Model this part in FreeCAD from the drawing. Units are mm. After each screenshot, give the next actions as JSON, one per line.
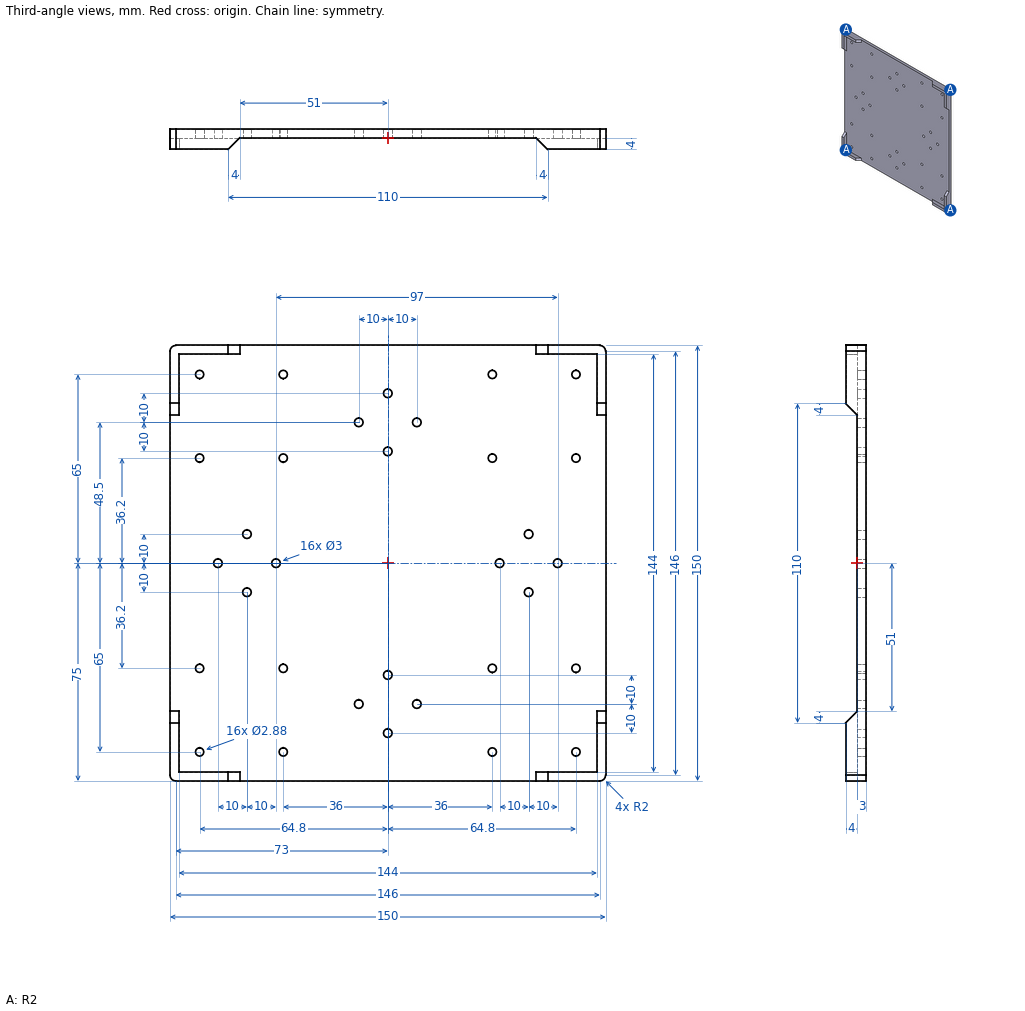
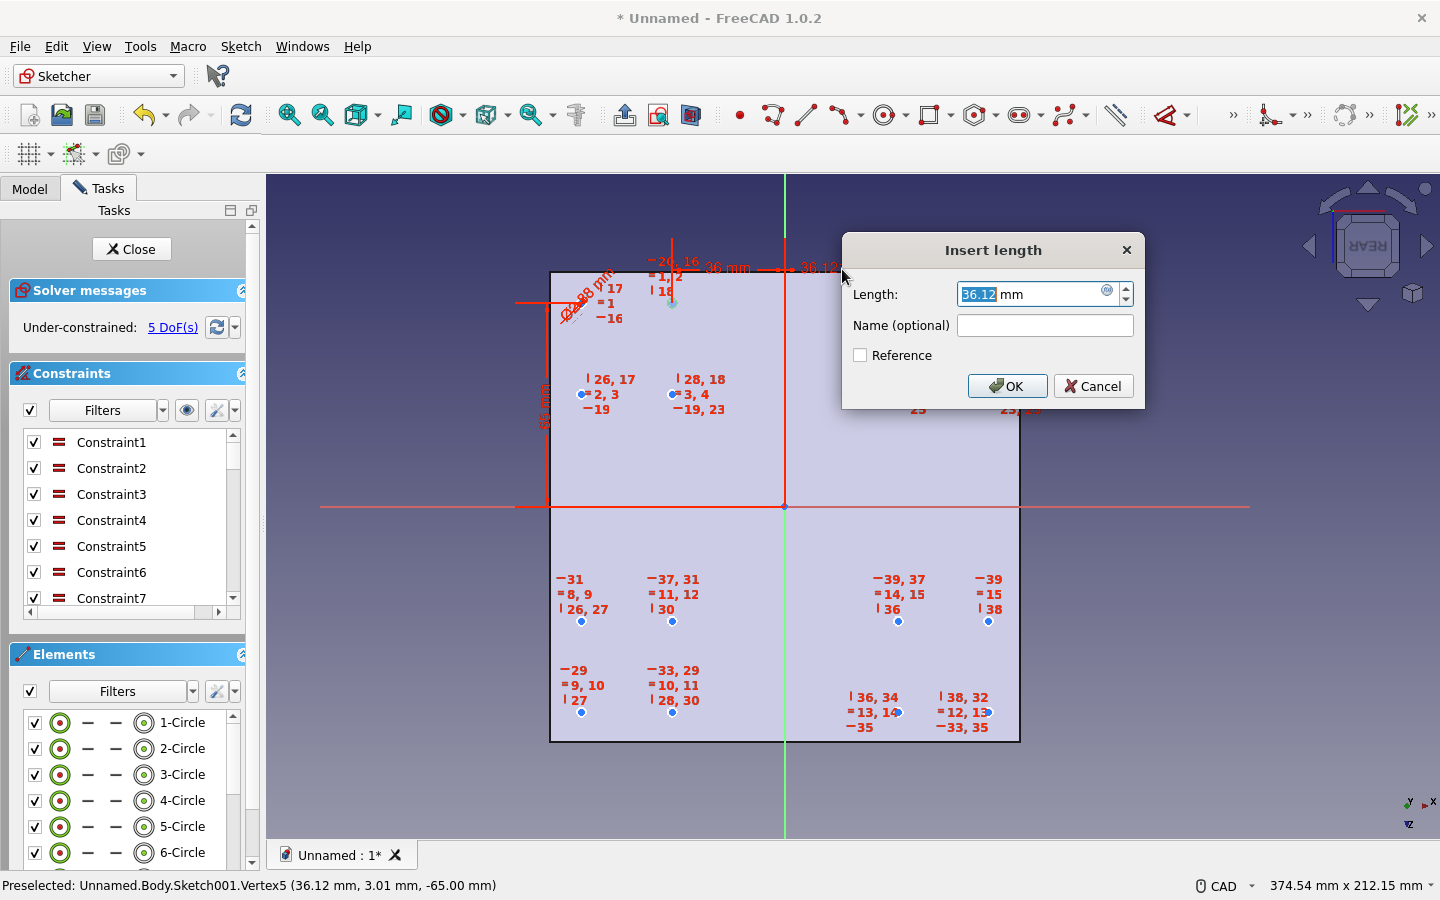
{"action": "type", "text": "36"}
{"action": "key", "text": "Return"}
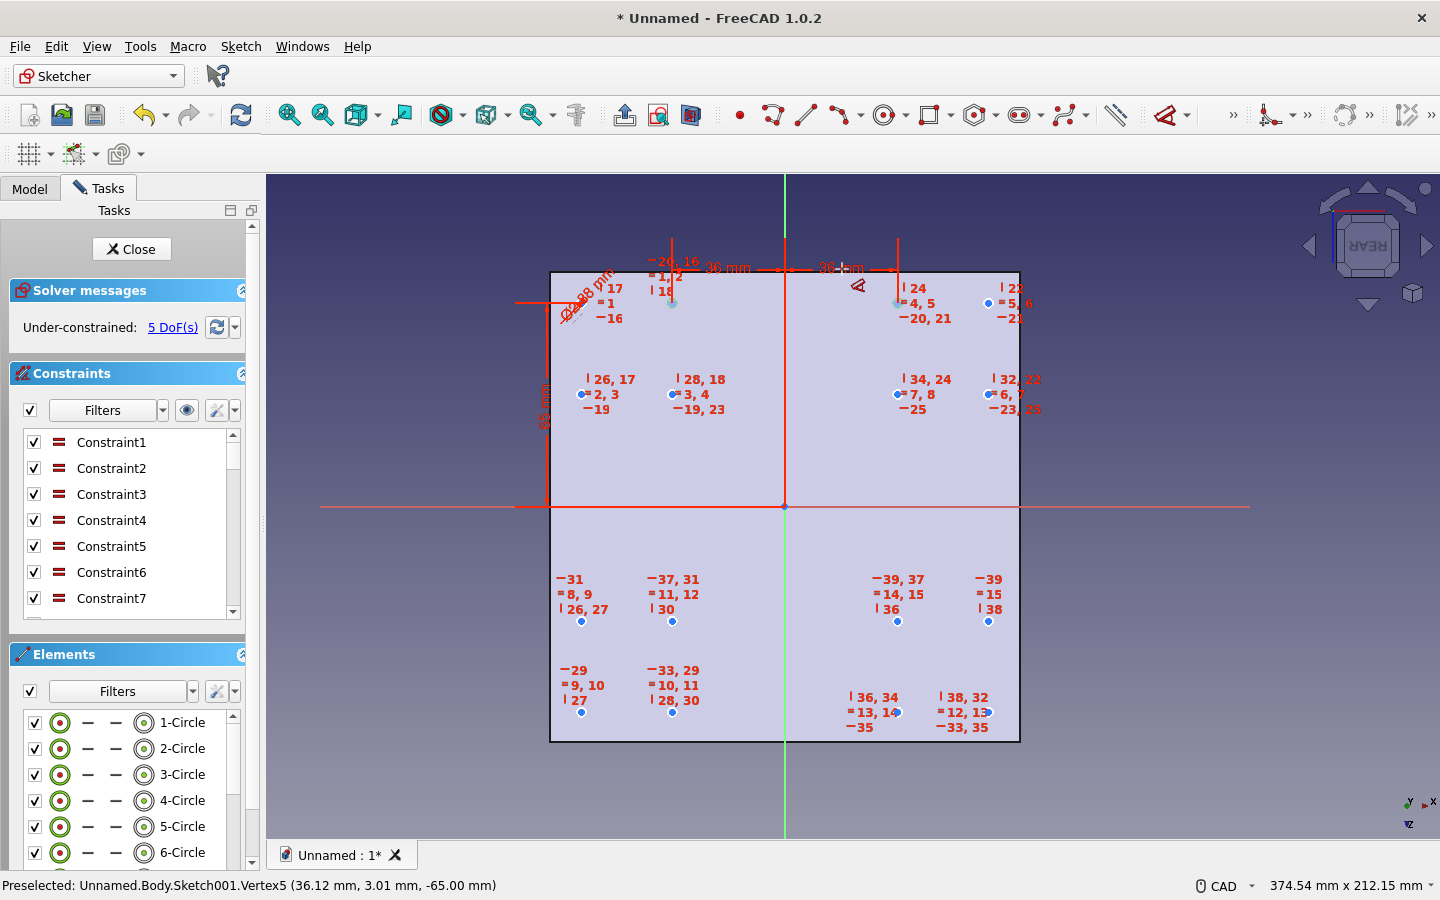
{"action": "left_click", "coordinate": [581, 712]}
{"action": "left_click", "coordinate": [547, 609]}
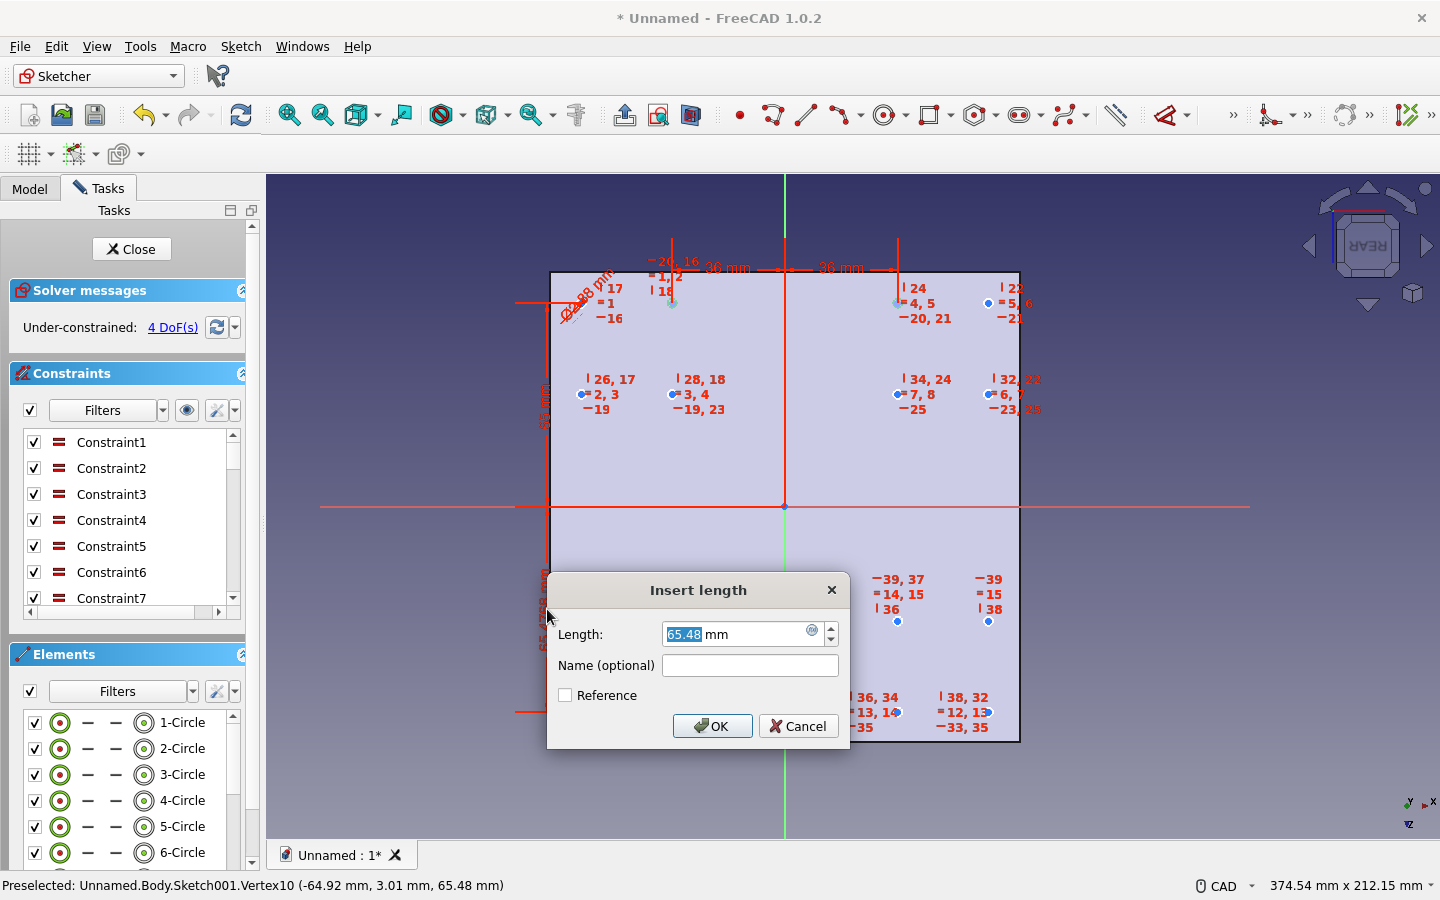
{"action": "type", "text": "65"}
{"action": "key", "text": "Return"}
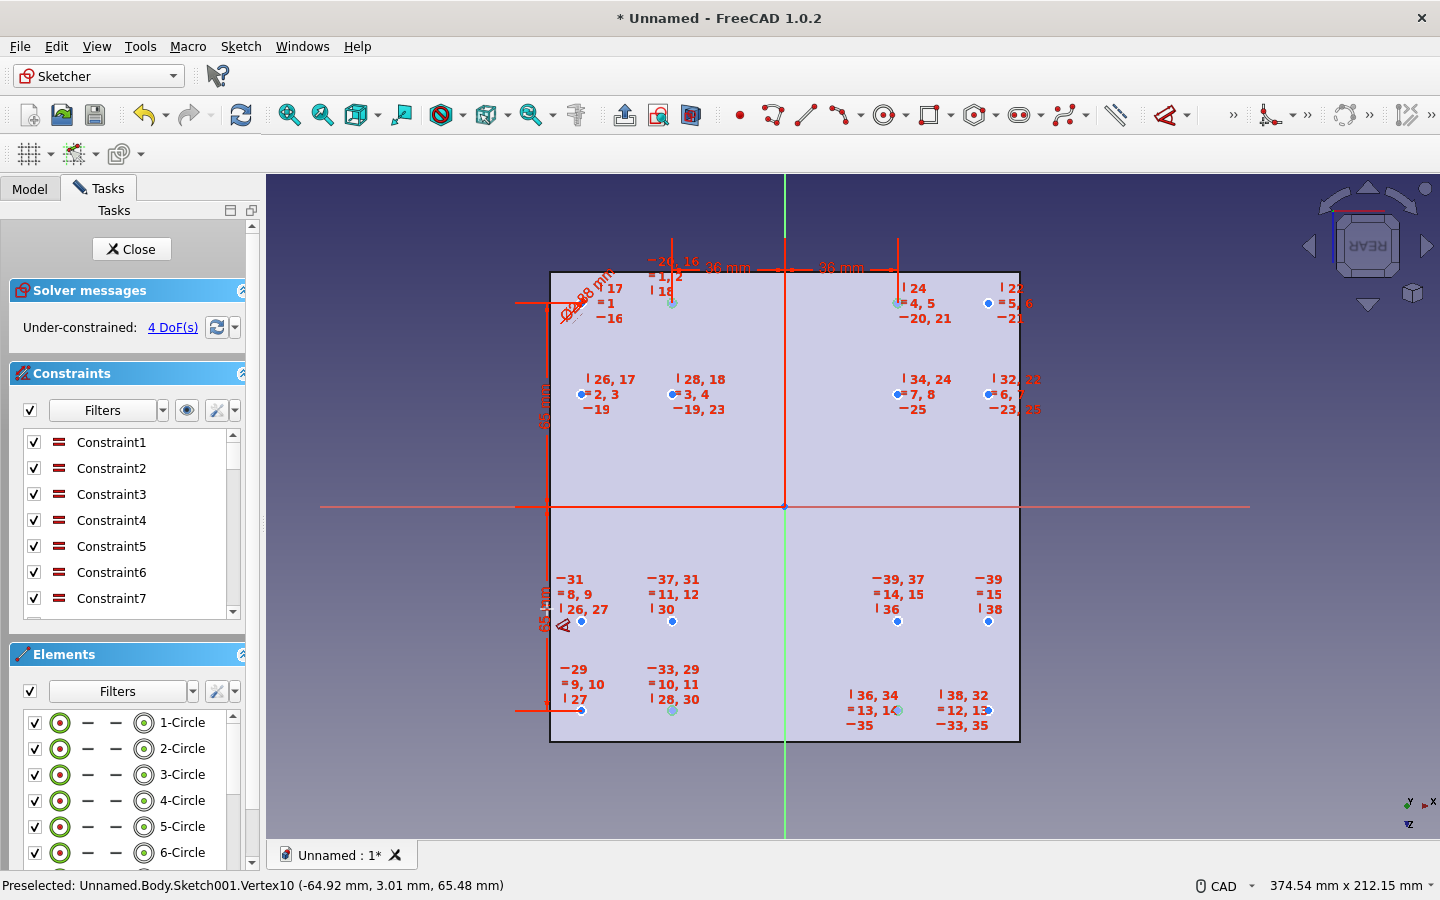
{"action": "left_click", "coordinate": [581, 303]}
{"action": "left_click", "coordinate": [636, 269]}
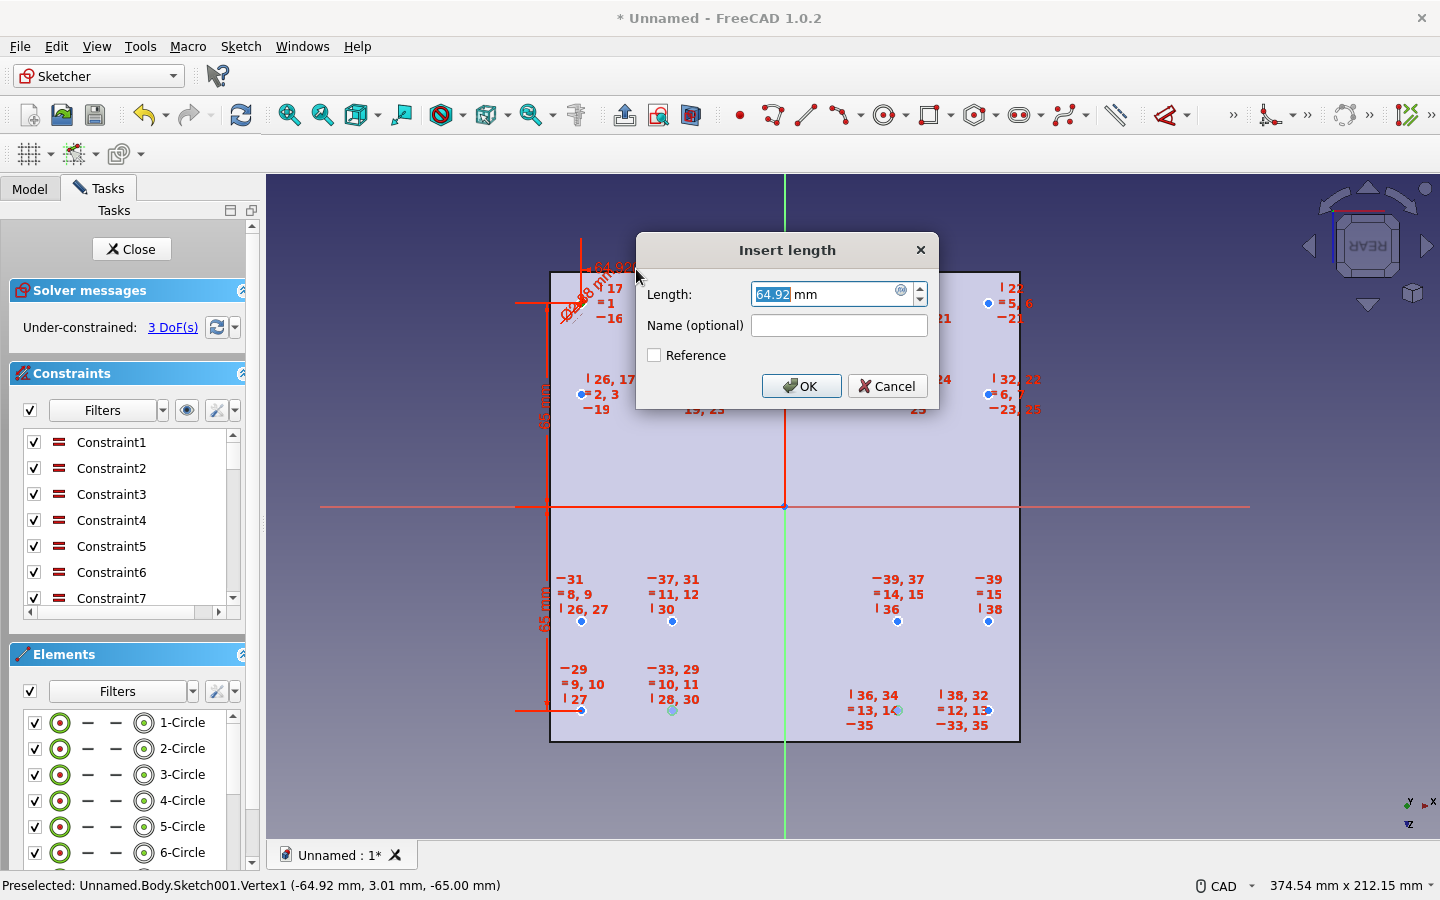
{"action": "type", "text": "64.8"}
{"action": "key", "text": "Return"}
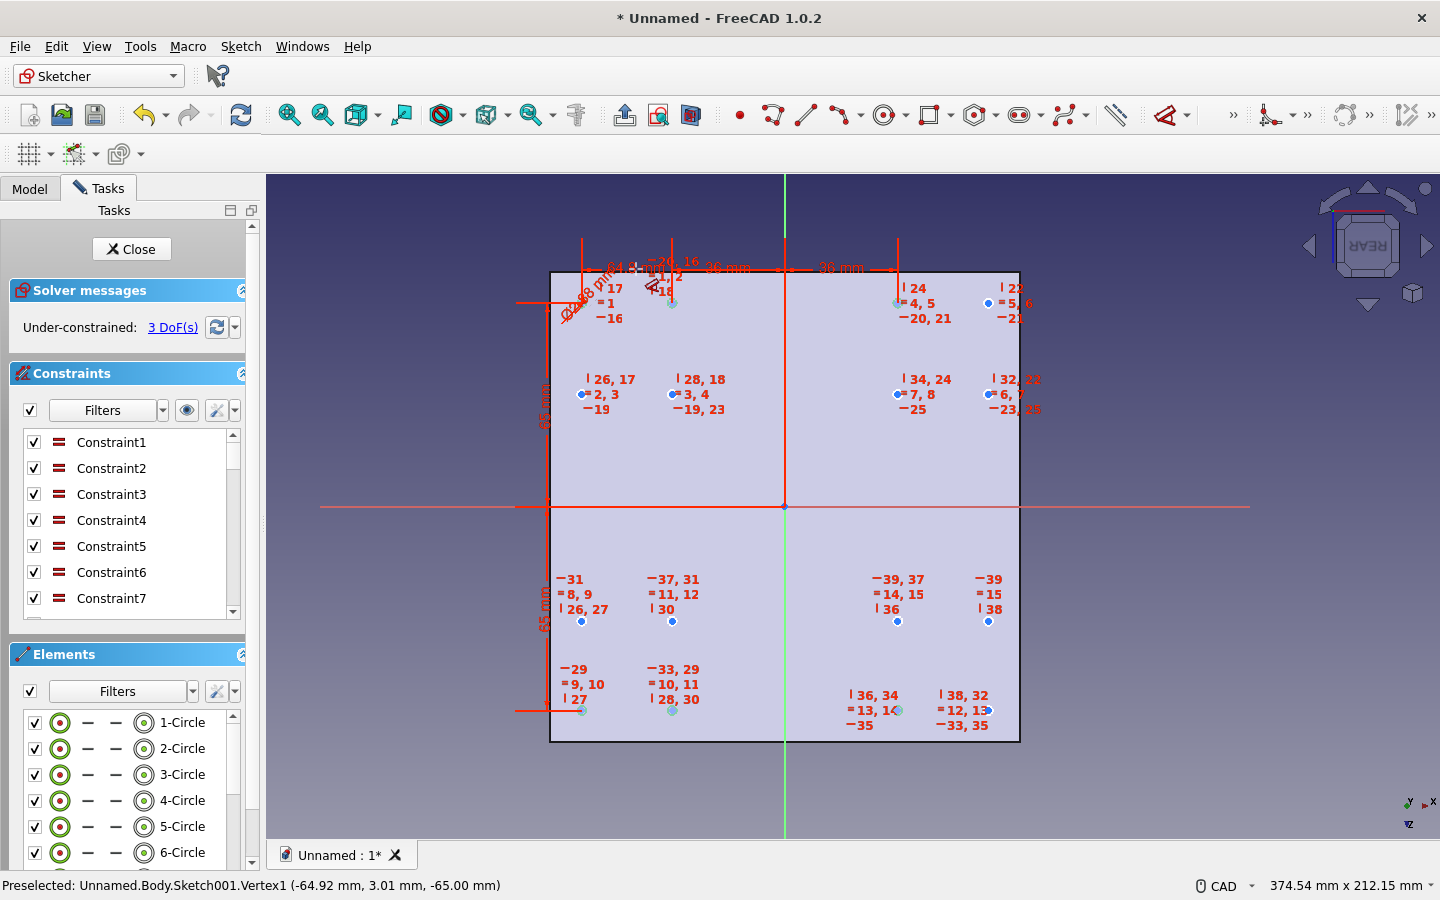
{"action": "left_click", "coordinate": [582, 394]}
{"action": "left_click", "coordinate": [548, 451]}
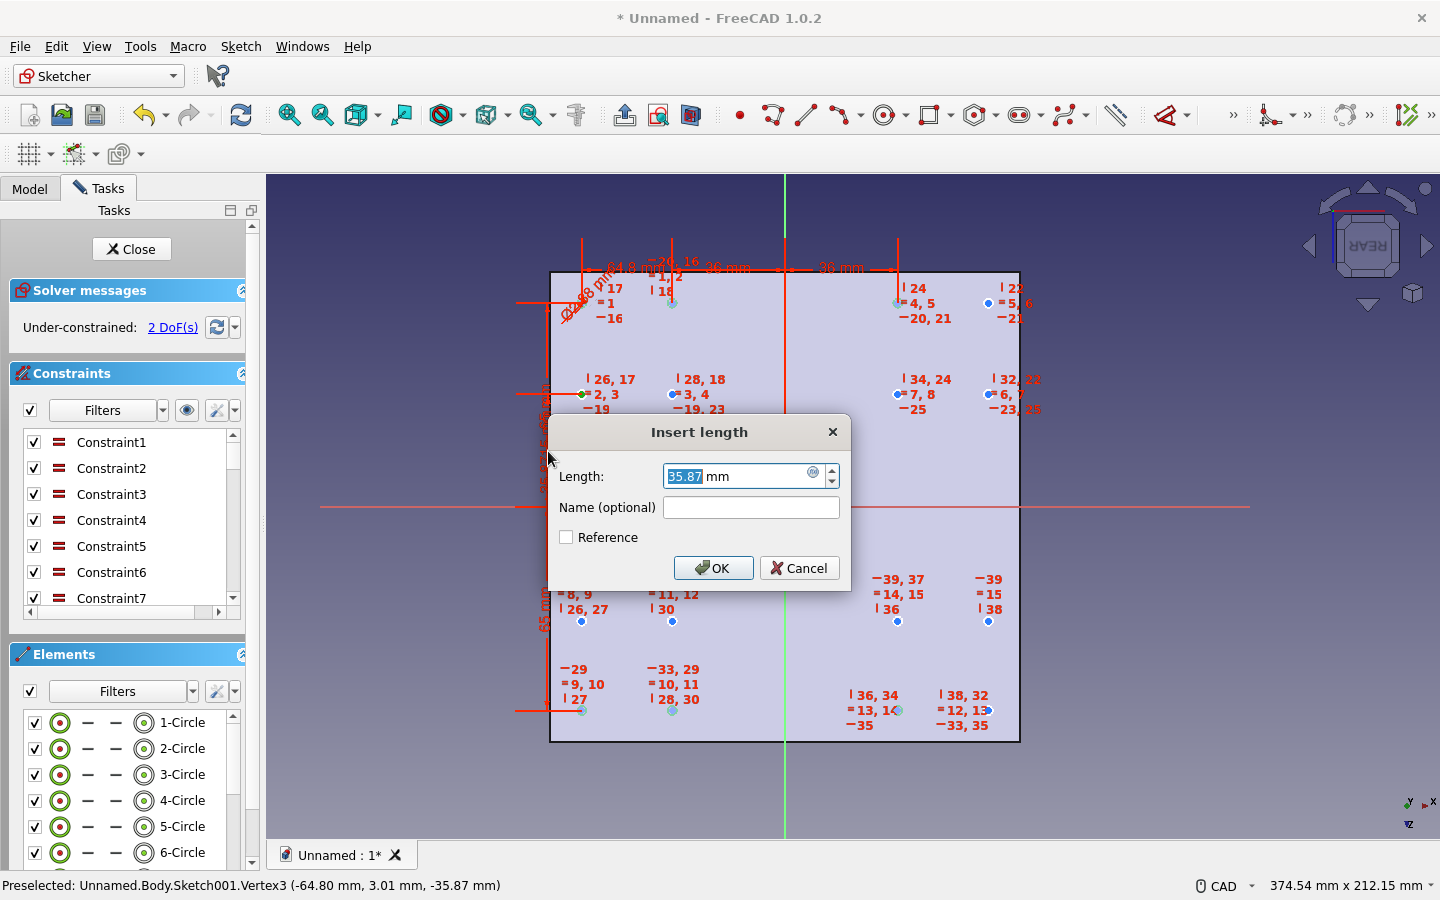
{"action": "type", "text": "36.2"}
{"action": "key", "text": "Return"}